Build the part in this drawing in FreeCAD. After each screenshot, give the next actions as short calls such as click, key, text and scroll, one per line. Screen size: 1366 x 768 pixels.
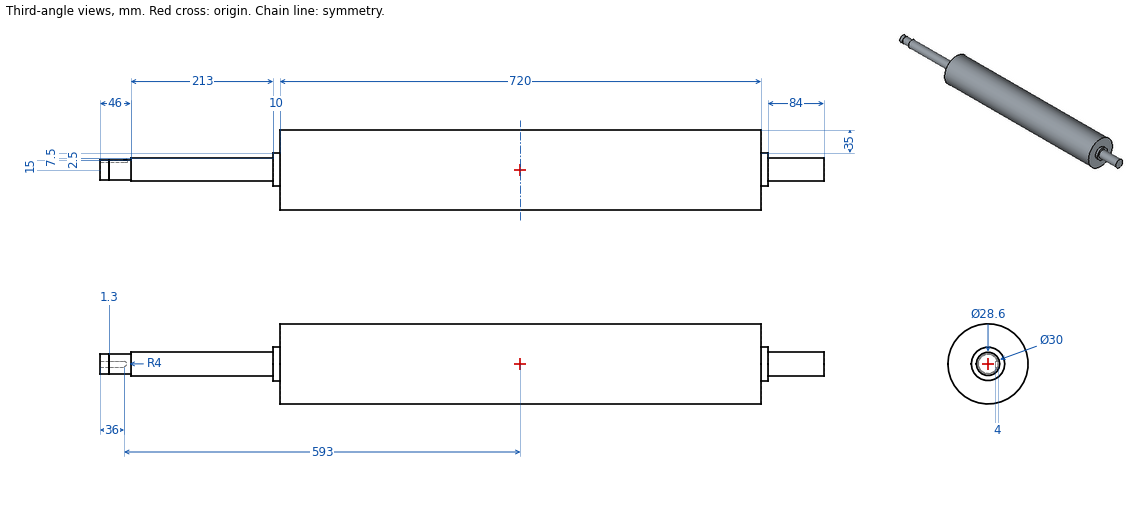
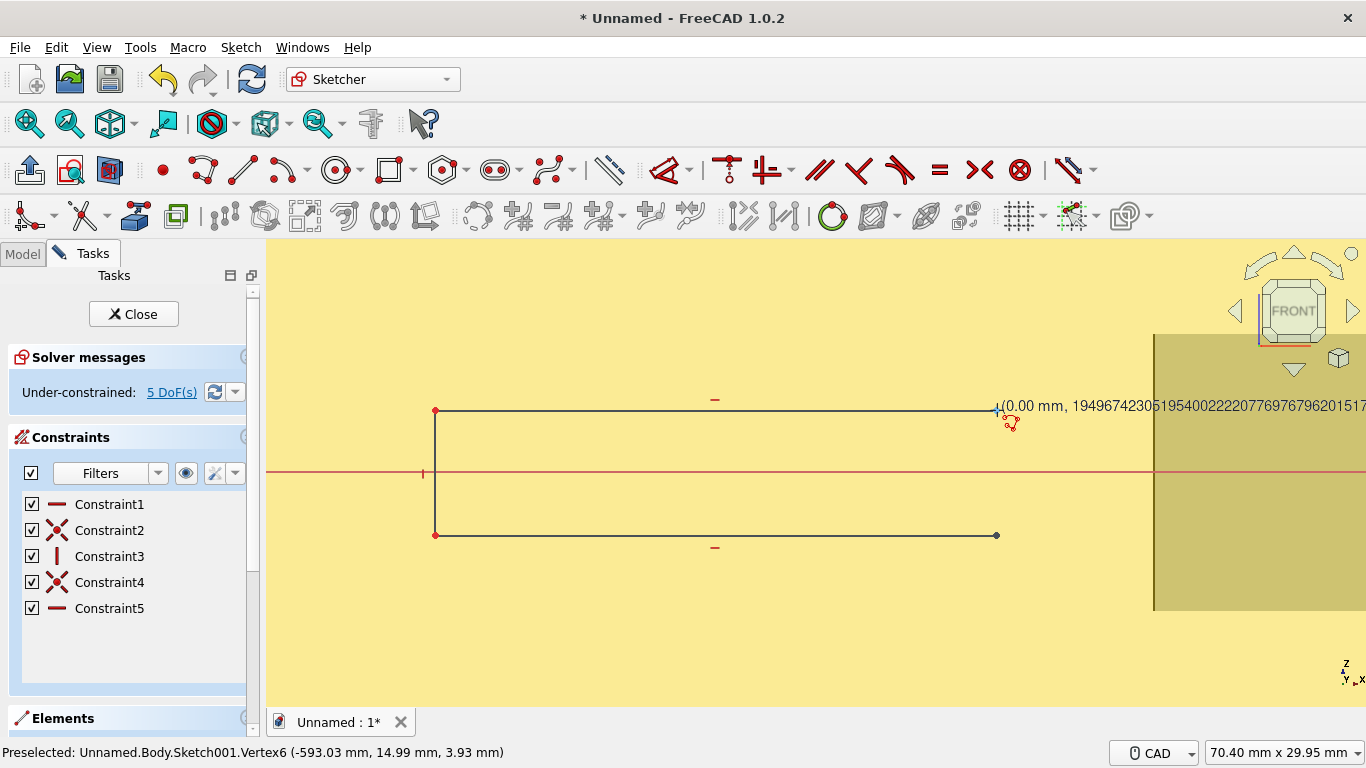
click(310, 170)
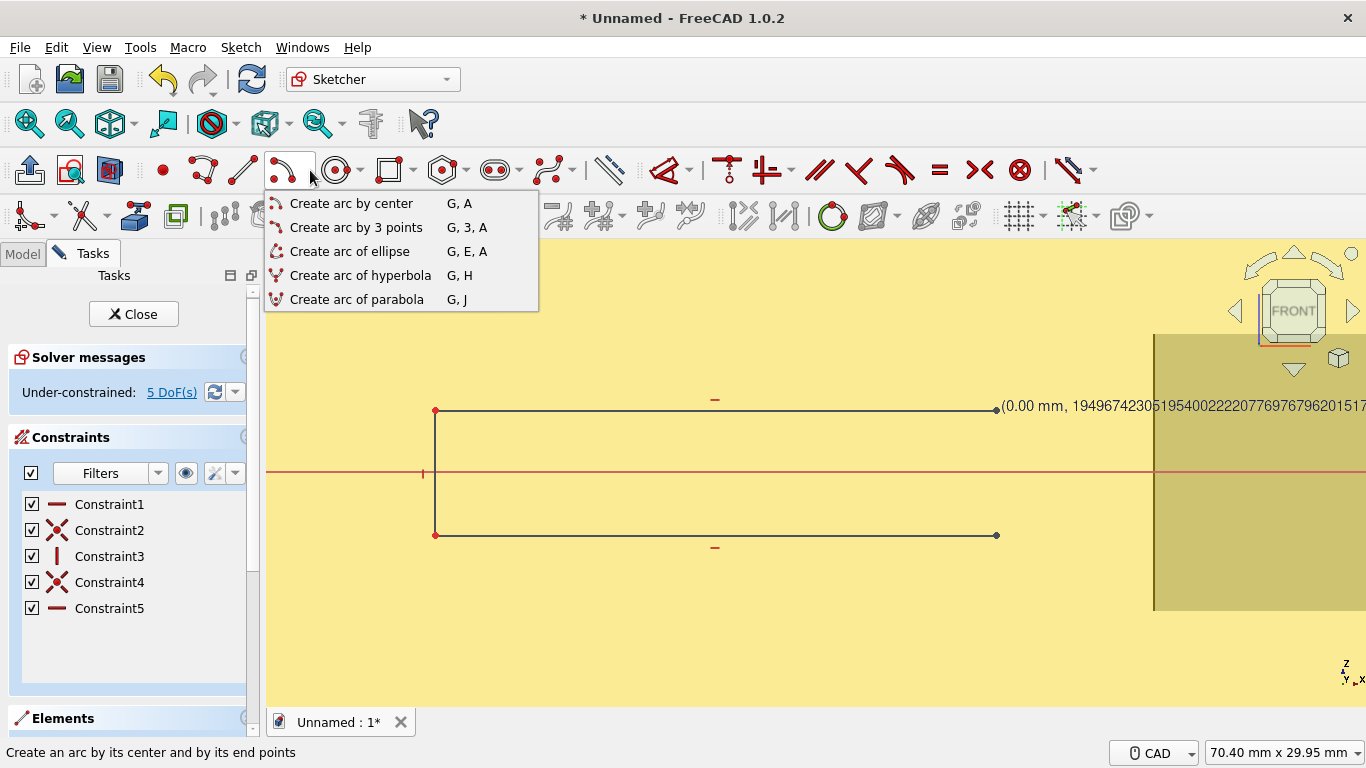
click(402, 227)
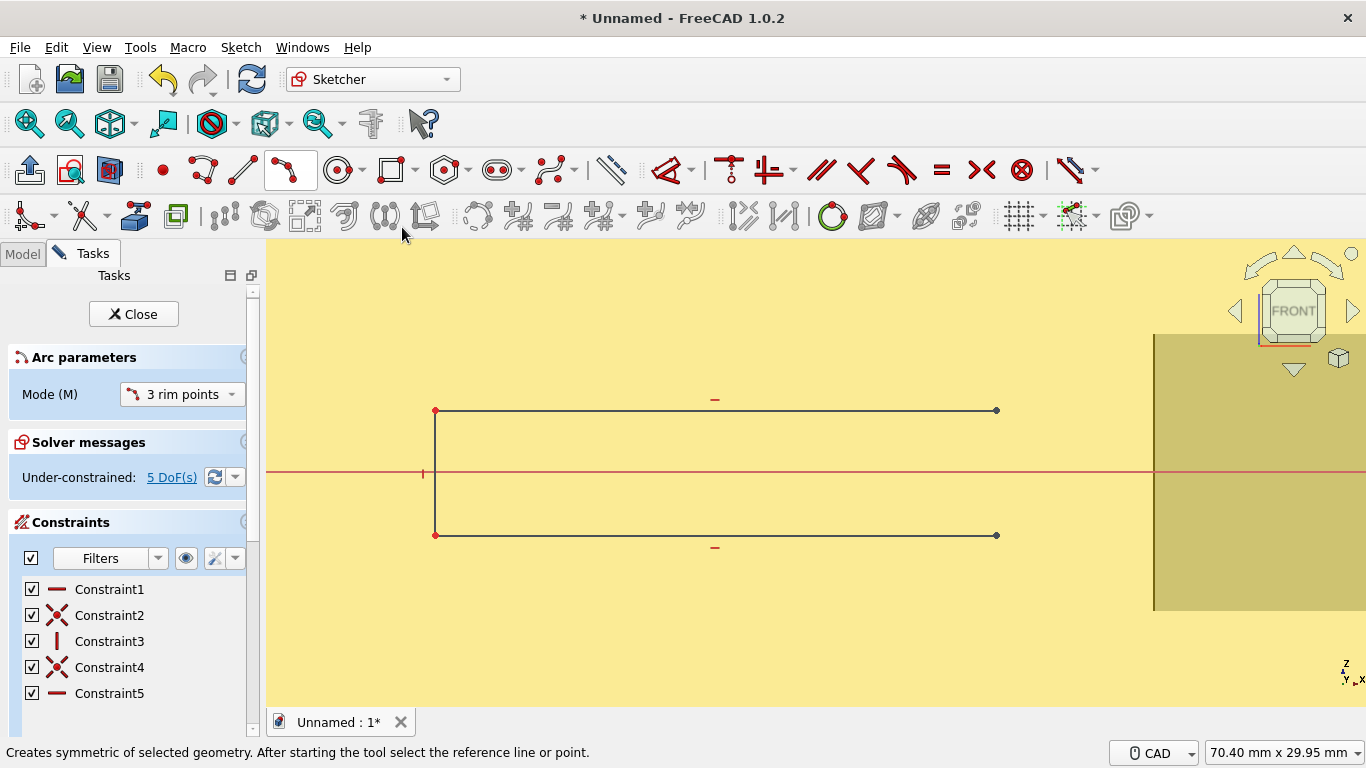
click(997, 411)
click(997, 536)
click(1057, 492)
key(Escape)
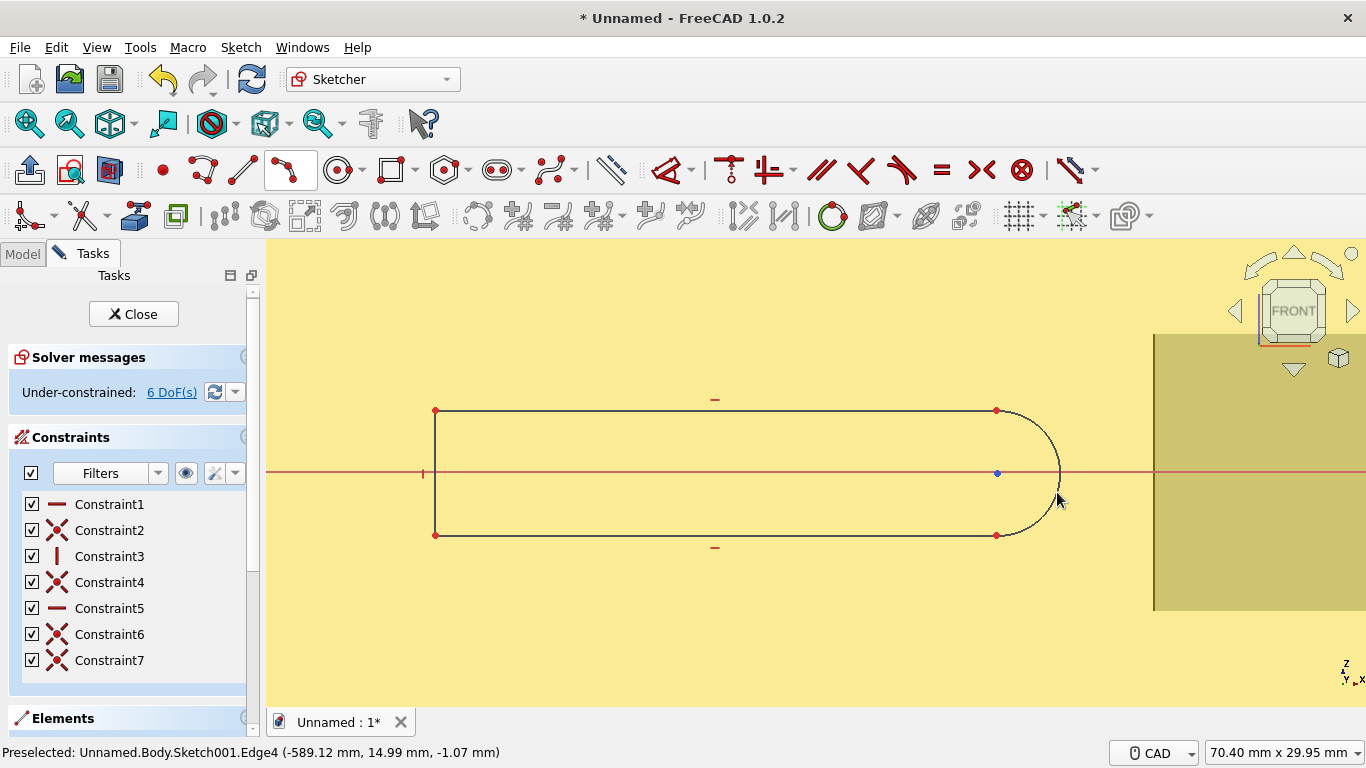
click(828, 536)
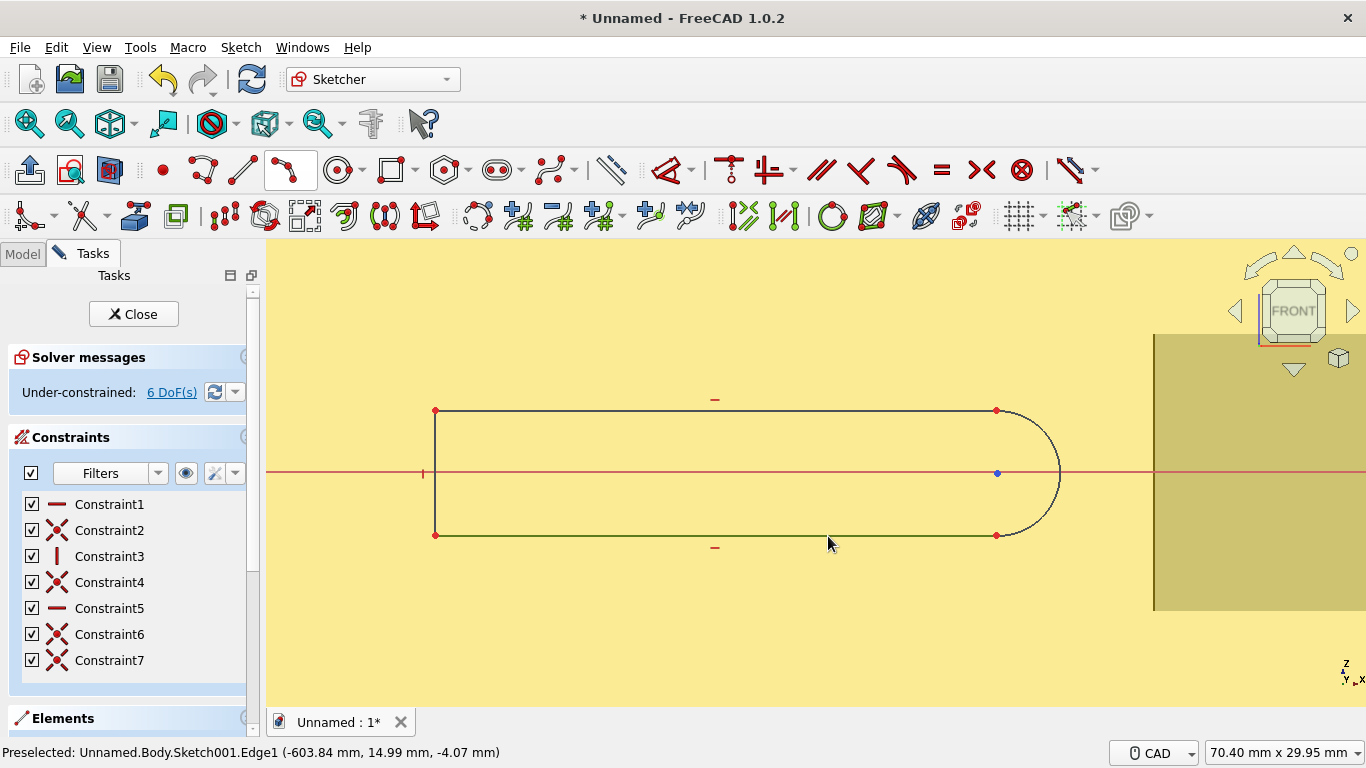
click(1048, 510)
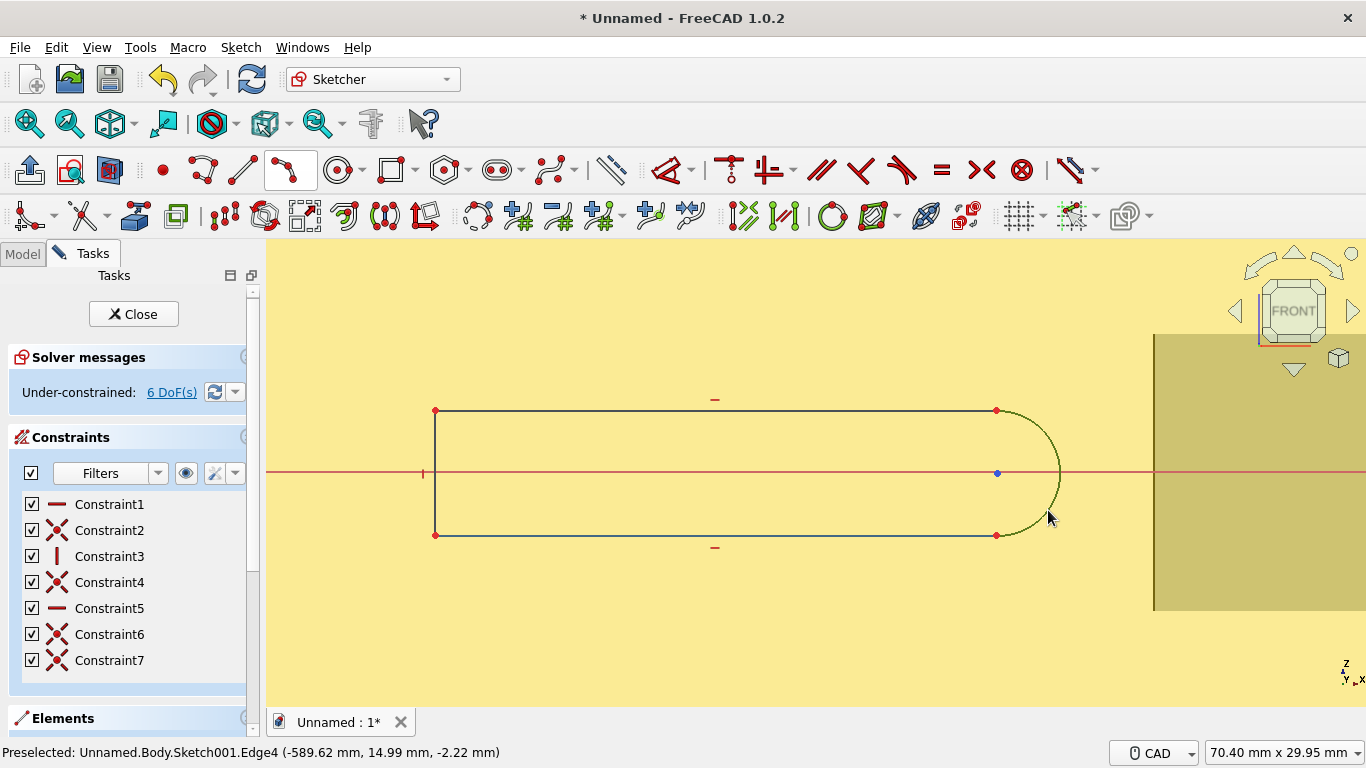
click(902, 170)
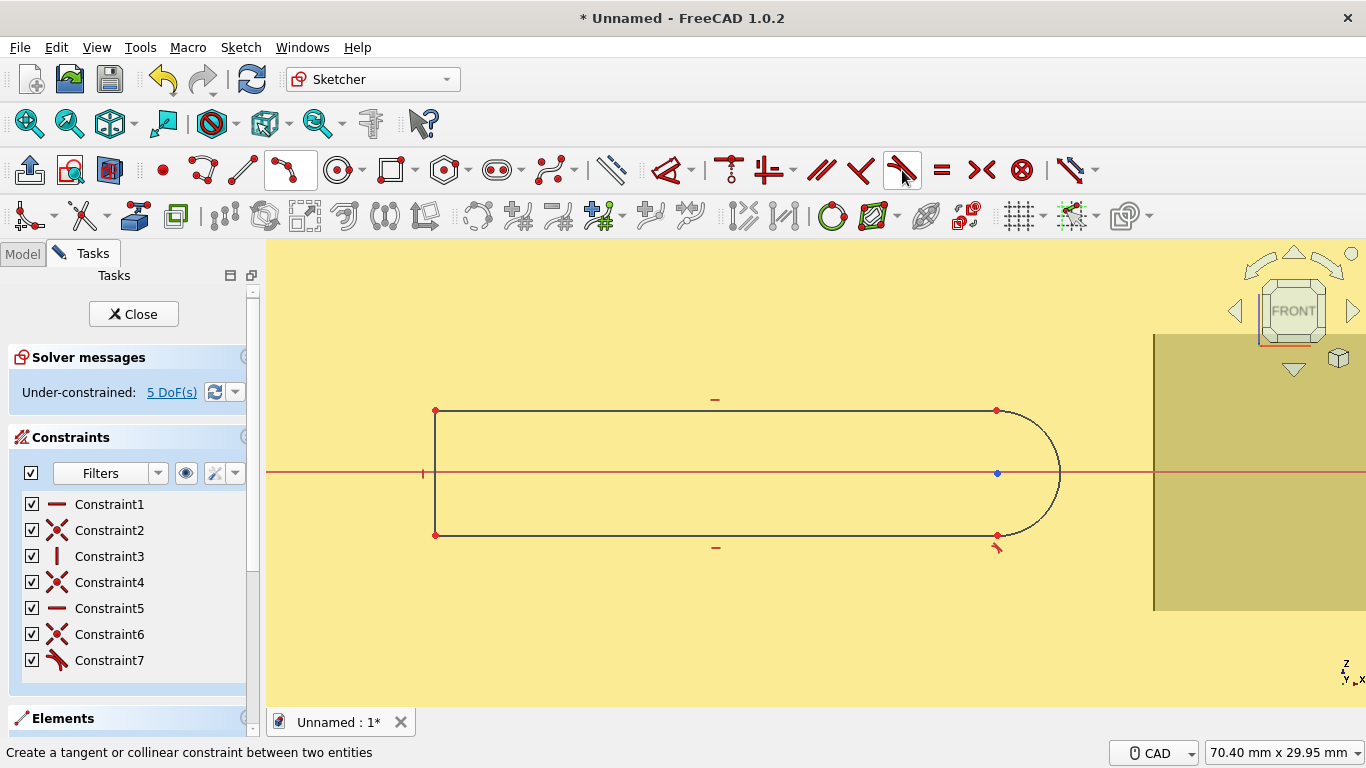
click(604, 411)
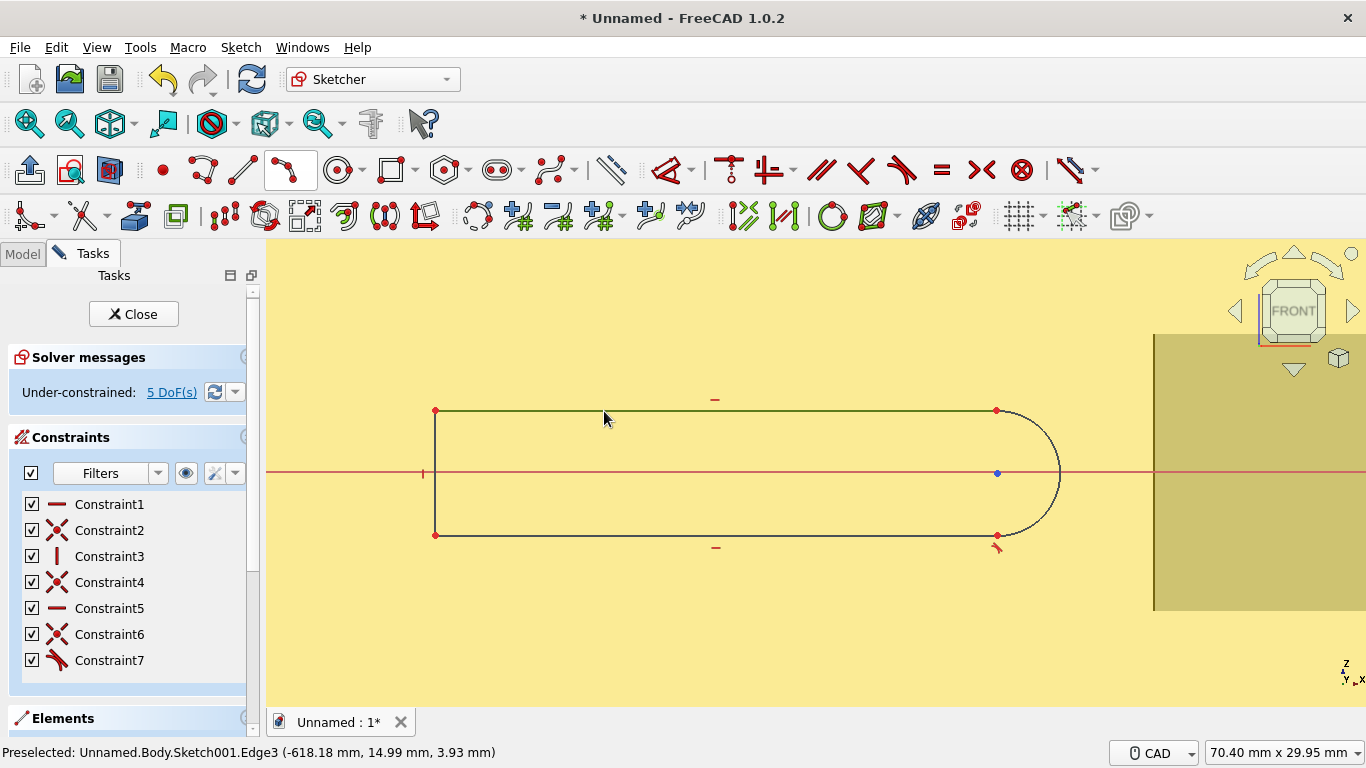
click(1048, 510)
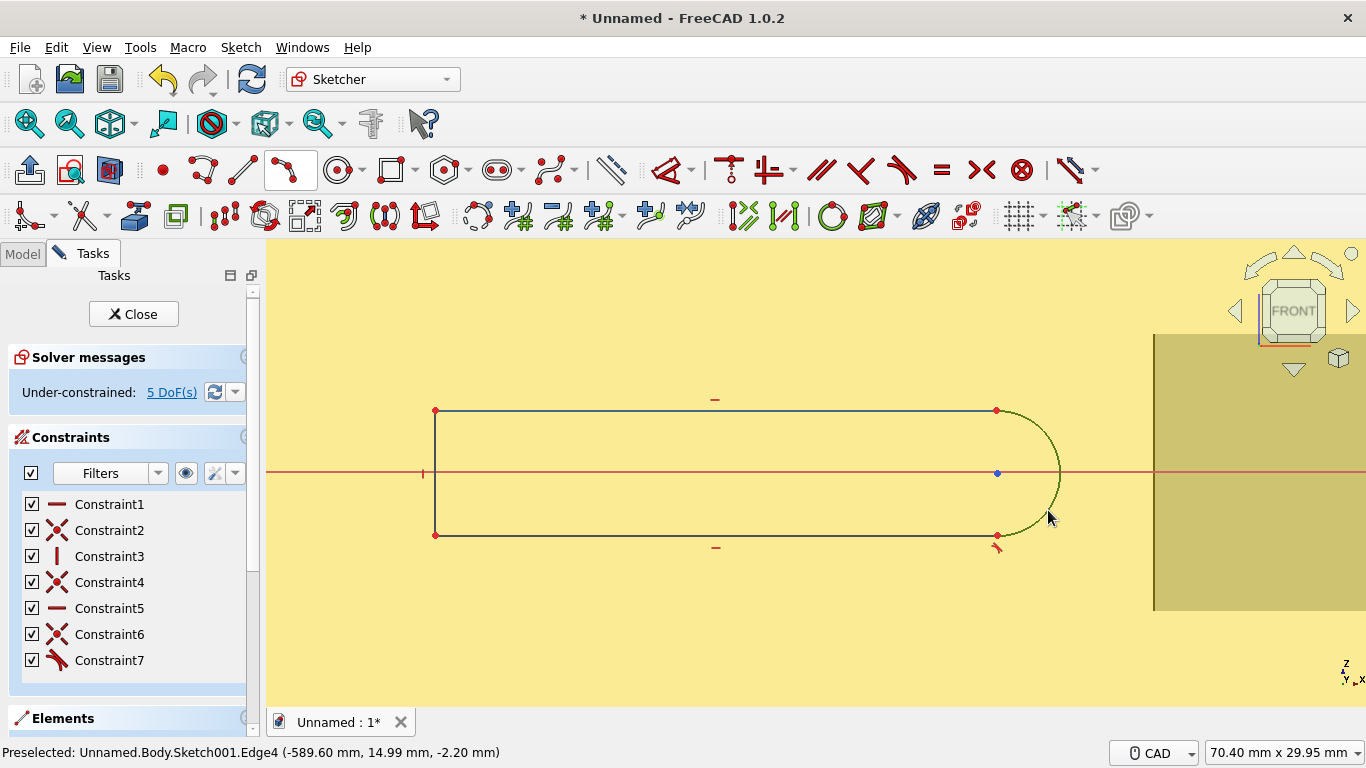
click(902, 170)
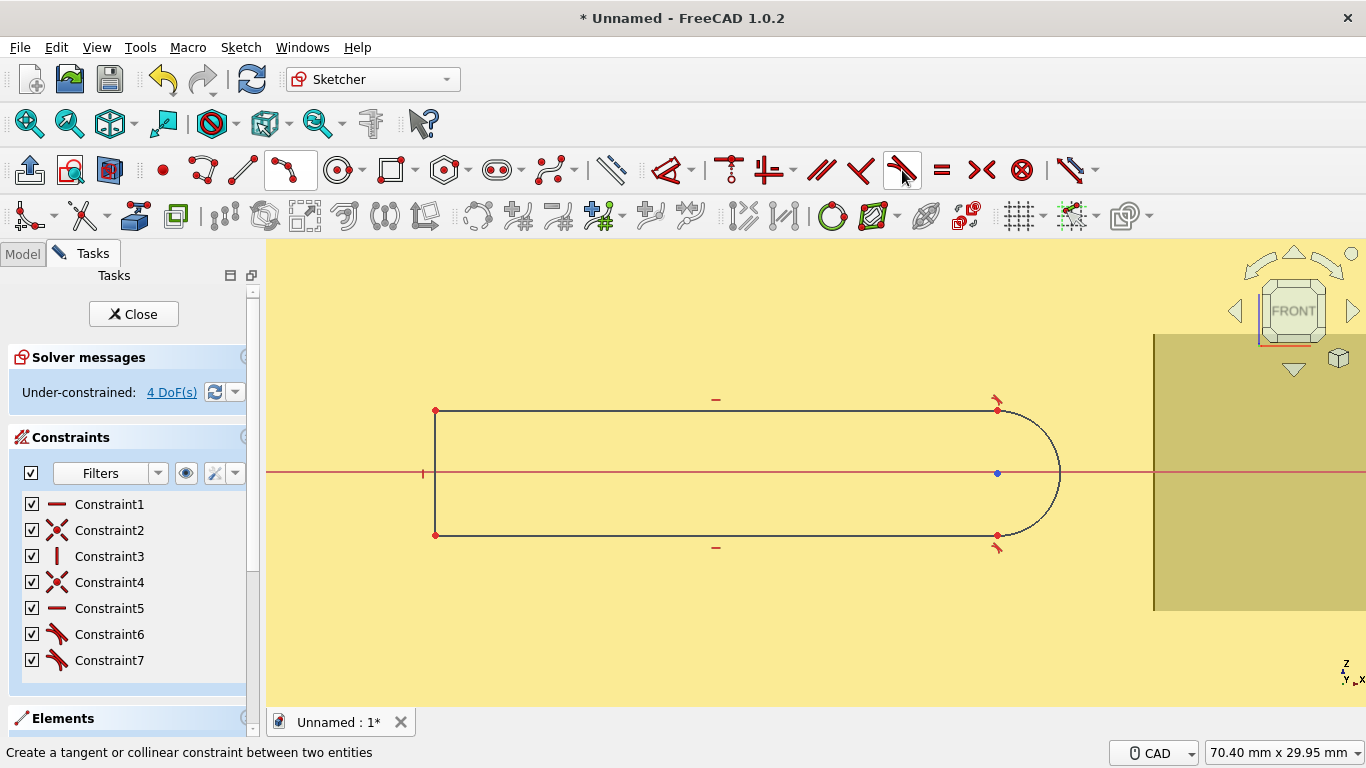
click(998, 474)